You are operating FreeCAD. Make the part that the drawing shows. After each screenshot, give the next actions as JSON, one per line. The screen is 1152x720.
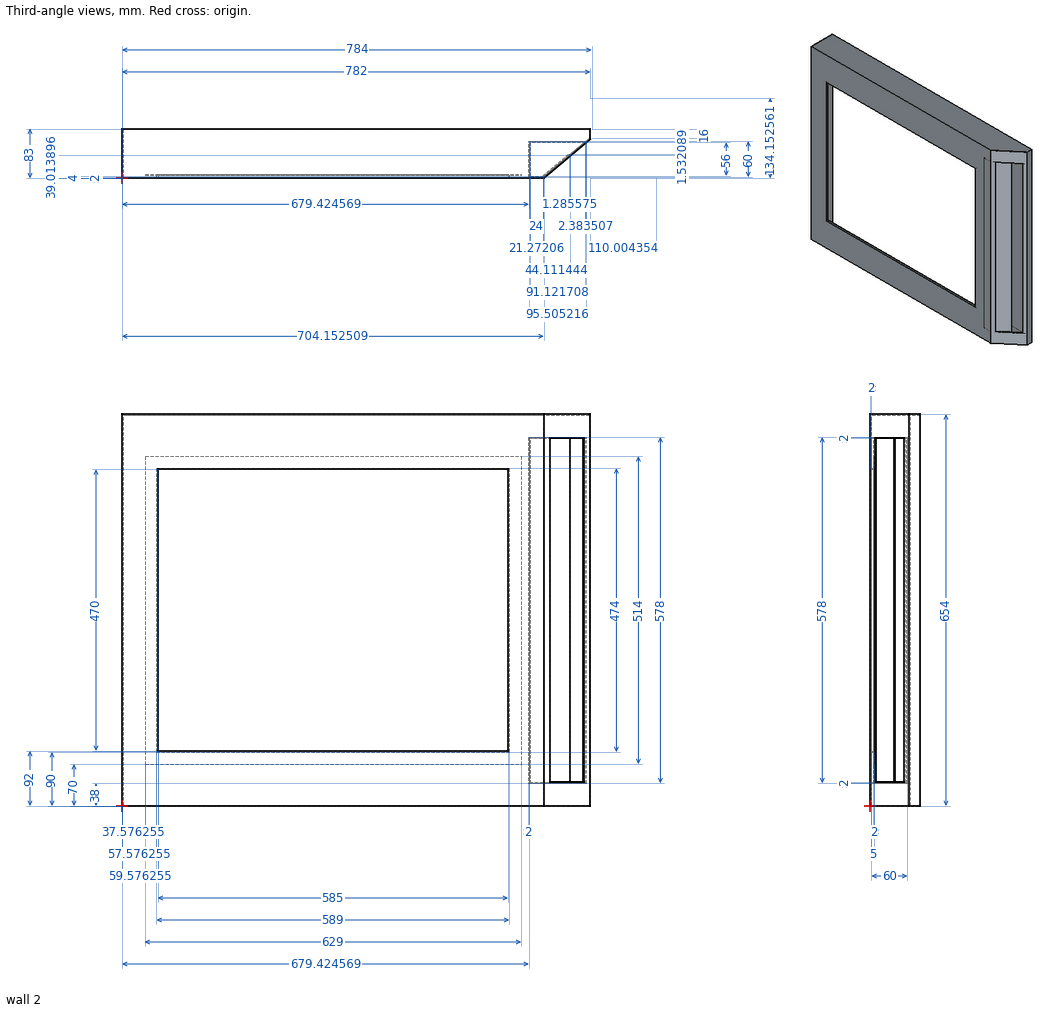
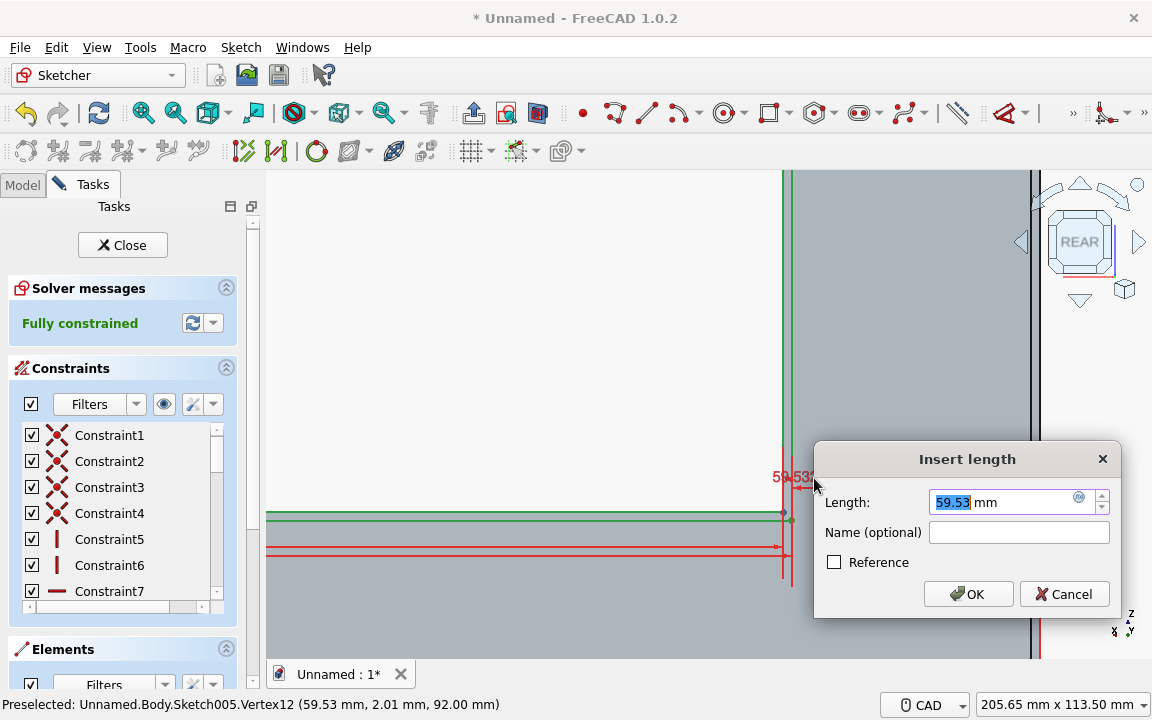
{"action": "type", "text": "59.576255"}
{"action": "key", "text": "Return"}
{"action": "key", "text": "Escape"}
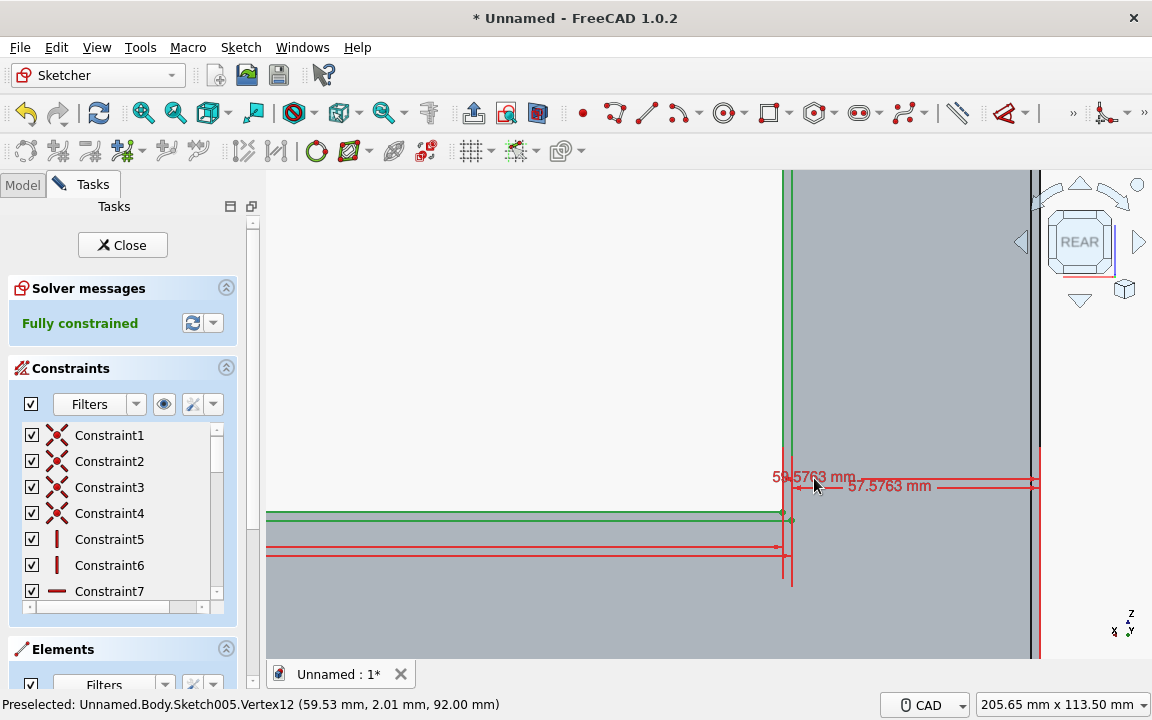
{"action": "left_click", "coordinate": [123, 245]}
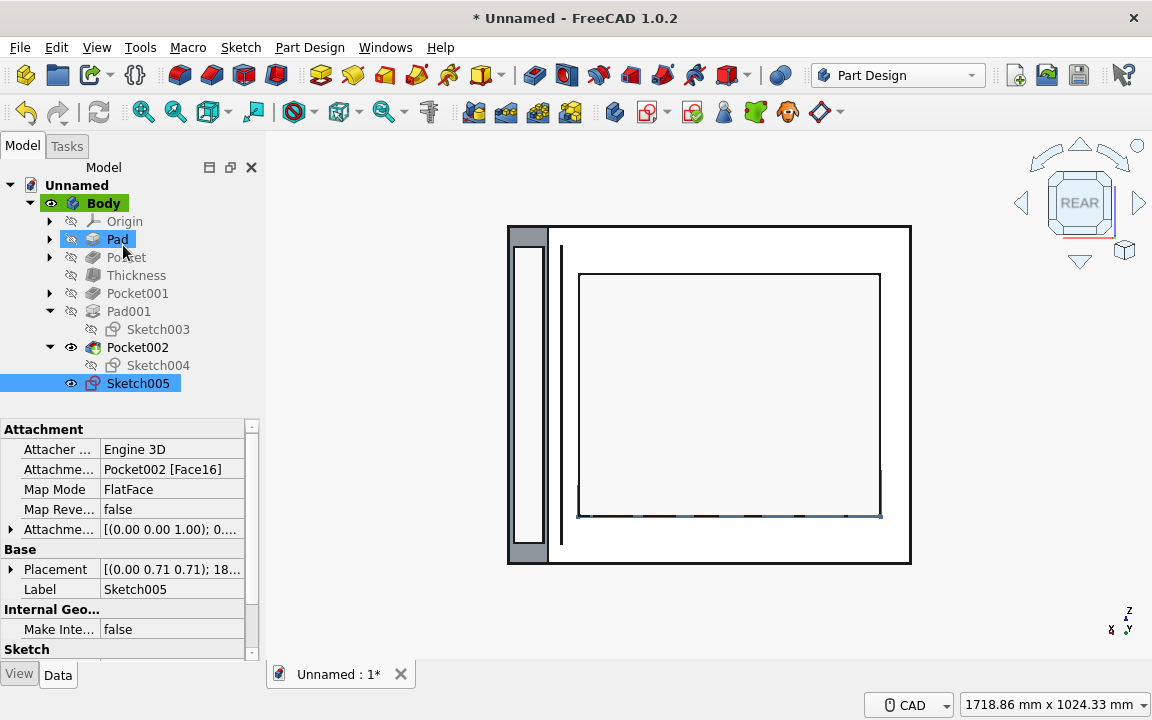
{"action": "left_click", "coordinate": [322, 76]}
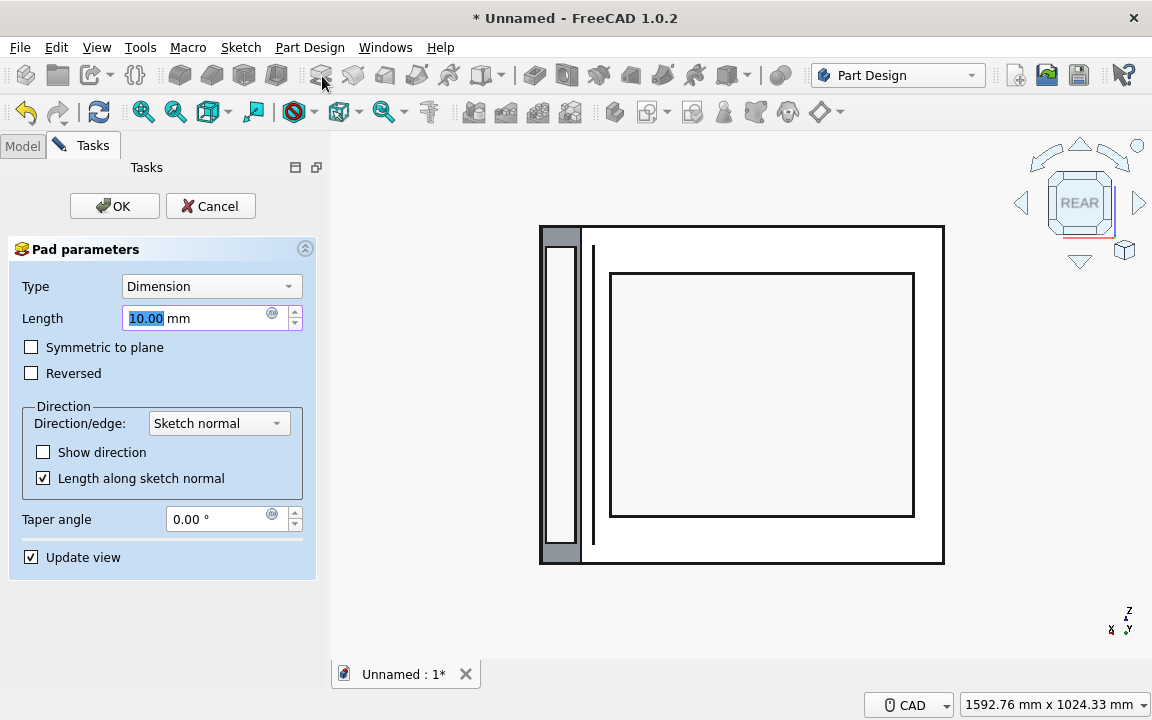
{"action": "type", "text": "5"}
{"action": "key", "text": "Tab"}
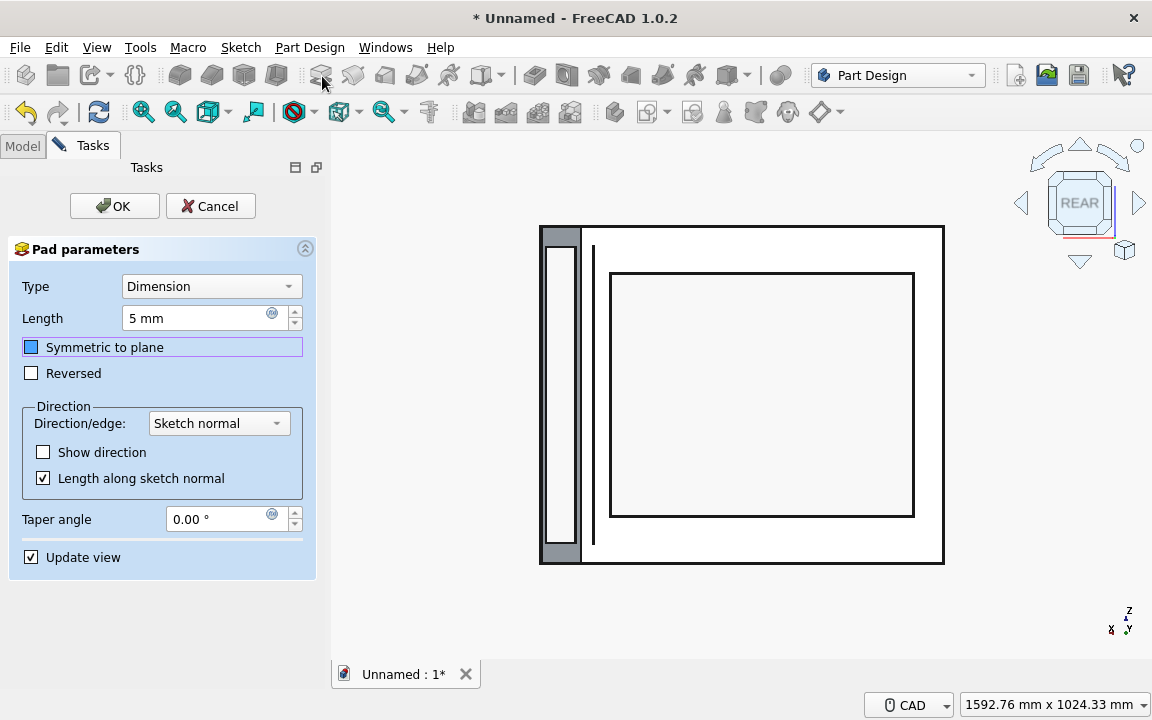
{"action": "left_click", "coordinate": [115, 206]}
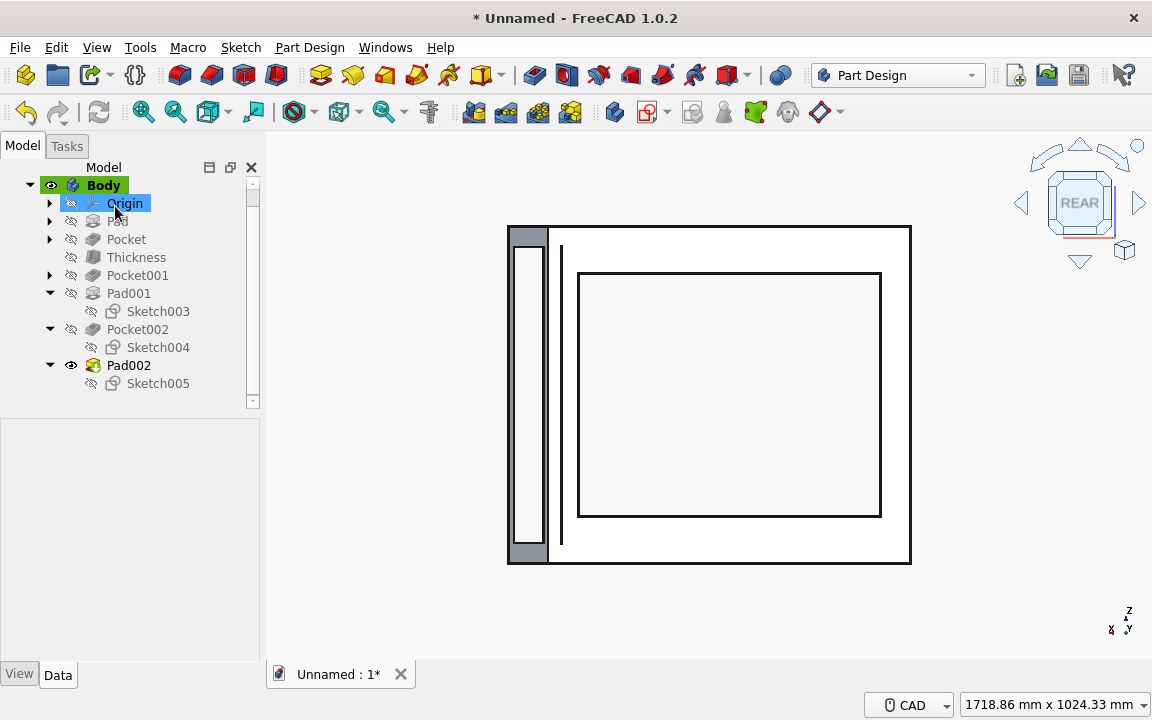
{"action": "scroll", "coordinate": [679, 516], "scroll_direction": "up", "scroll_amount": 15}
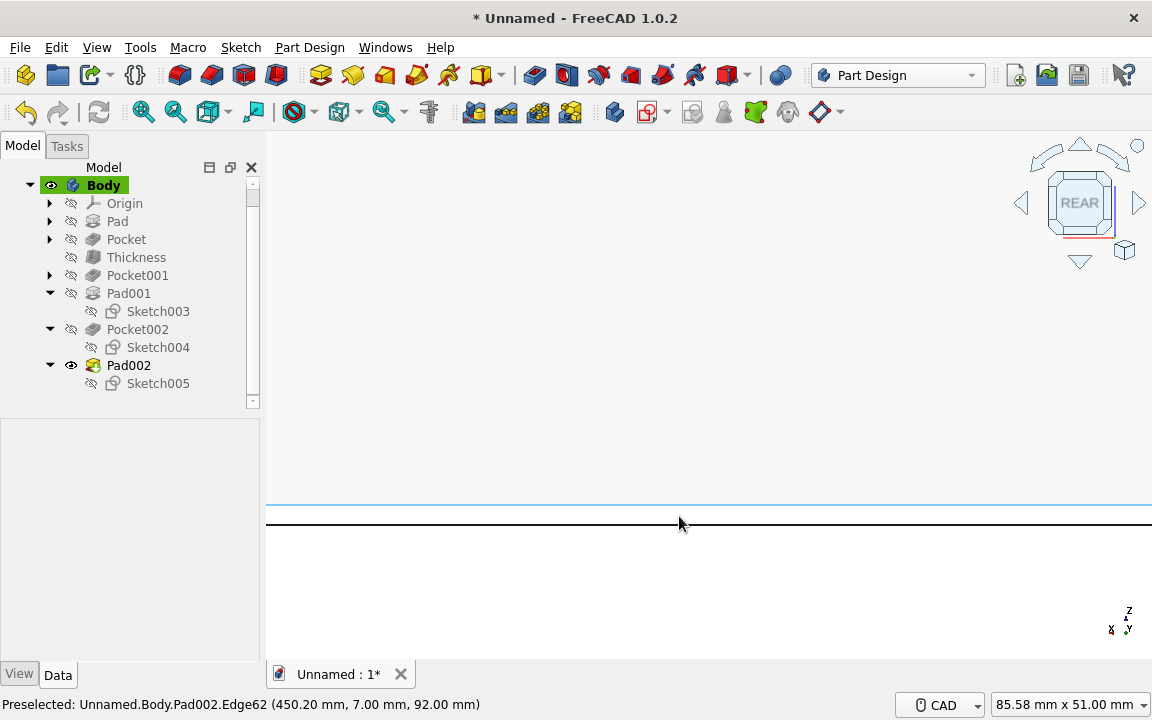
{"action": "scroll", "coordinate": [677, 518], "scroll_direction": "up", "scroll_amount": 3}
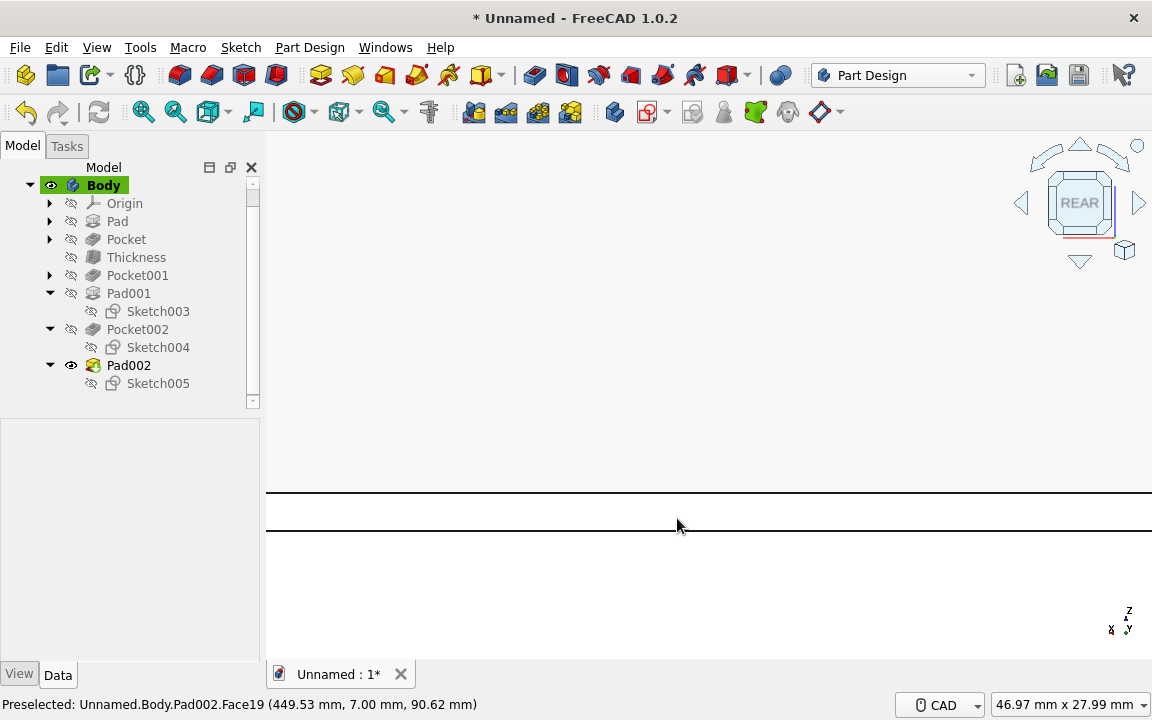
{"action": "left_click", "coordinate": [676, 517]}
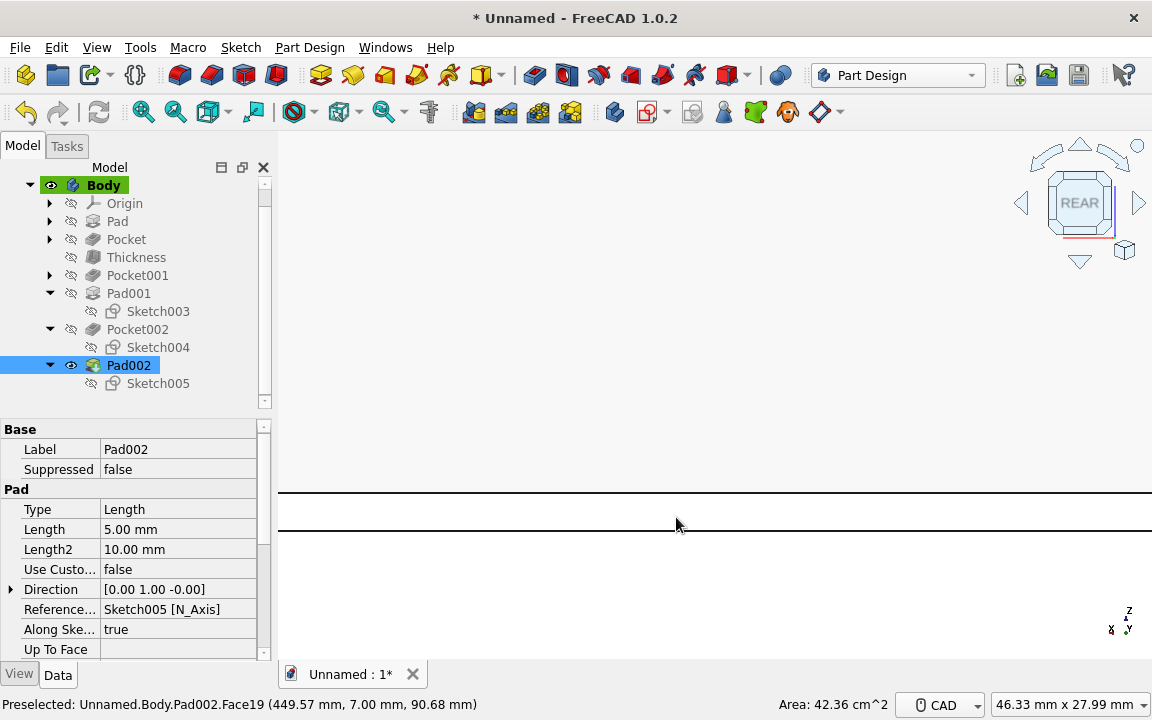
{"action": "left_click", "coordinate": [648, 112]}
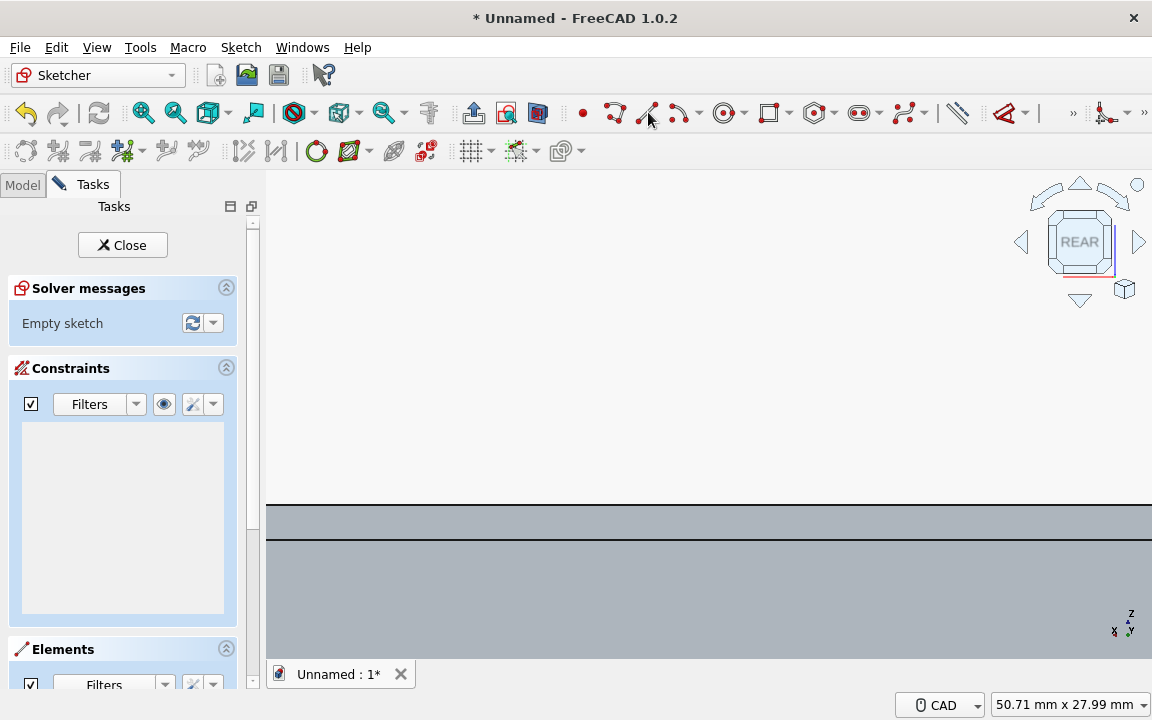
{"action": "key", "text": "q s"}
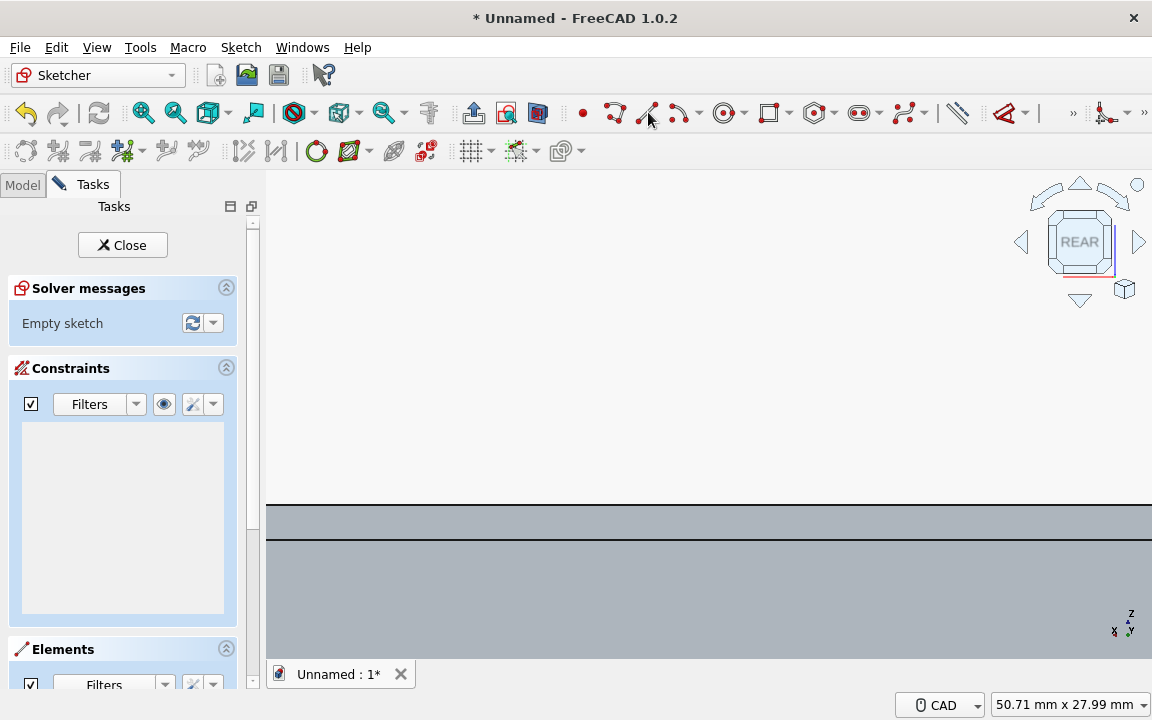
{"action": "scroll", "coordinate": [569, 532], "scroll_direction": "down", "scroll_amount": 17}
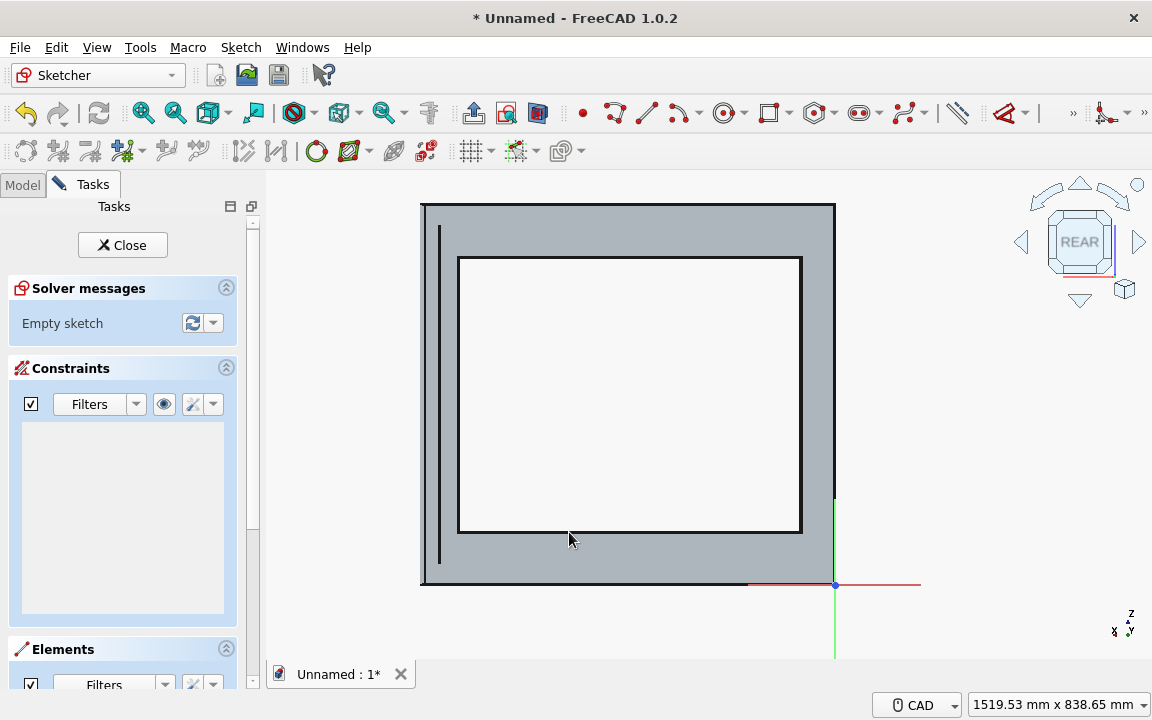
{"action": "key", "text": "g r"}